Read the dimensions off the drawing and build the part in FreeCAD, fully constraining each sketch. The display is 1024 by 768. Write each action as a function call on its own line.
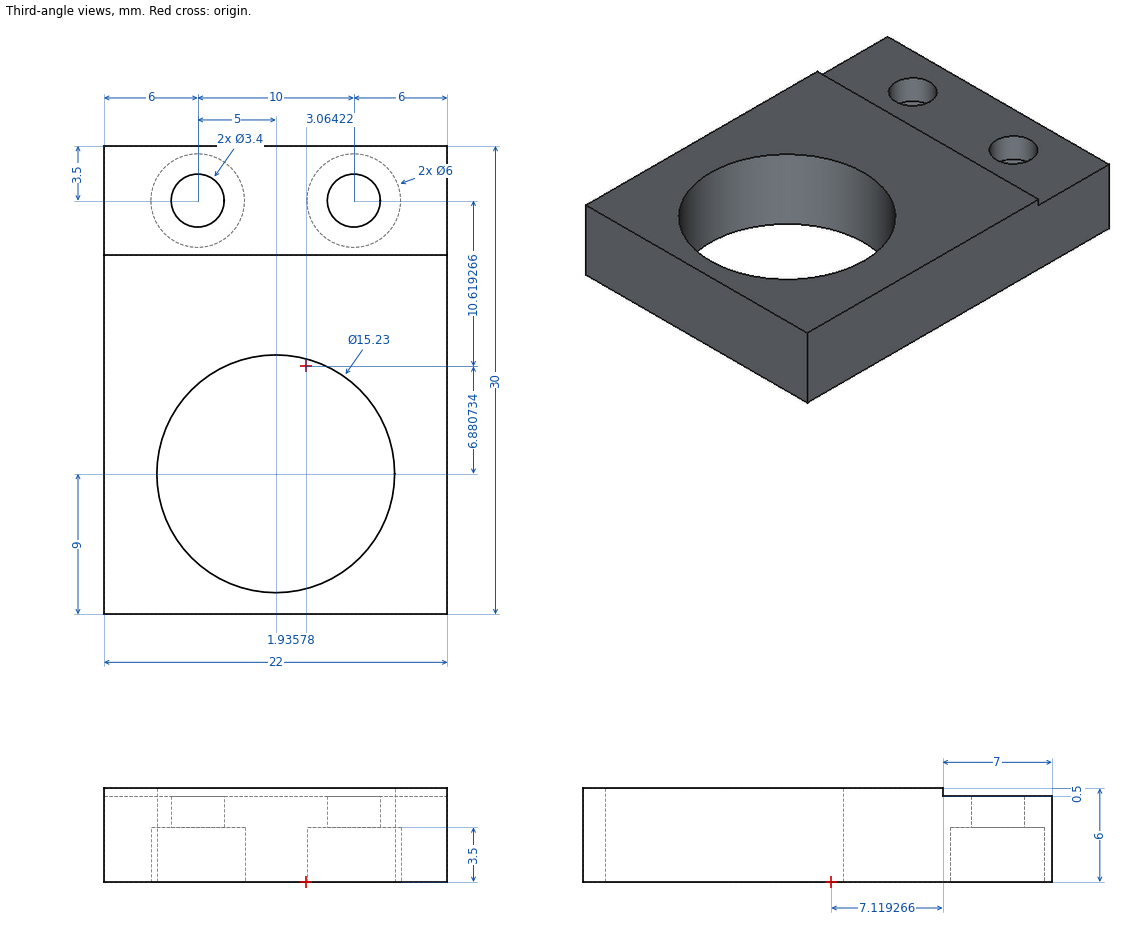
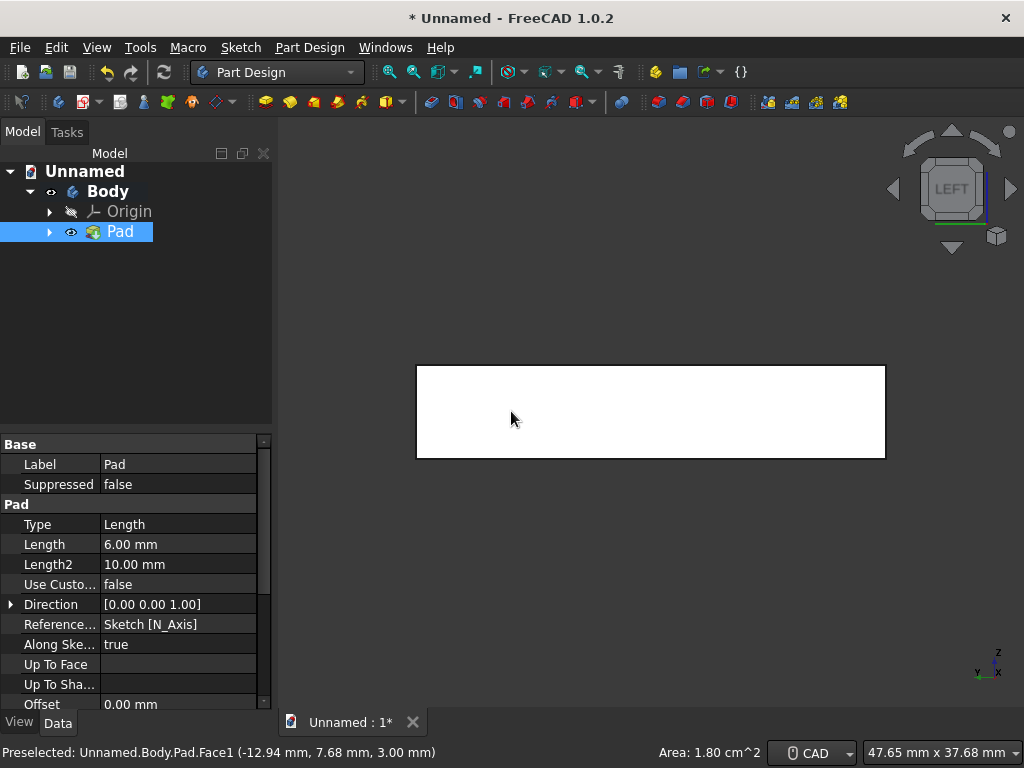
click(84, 102)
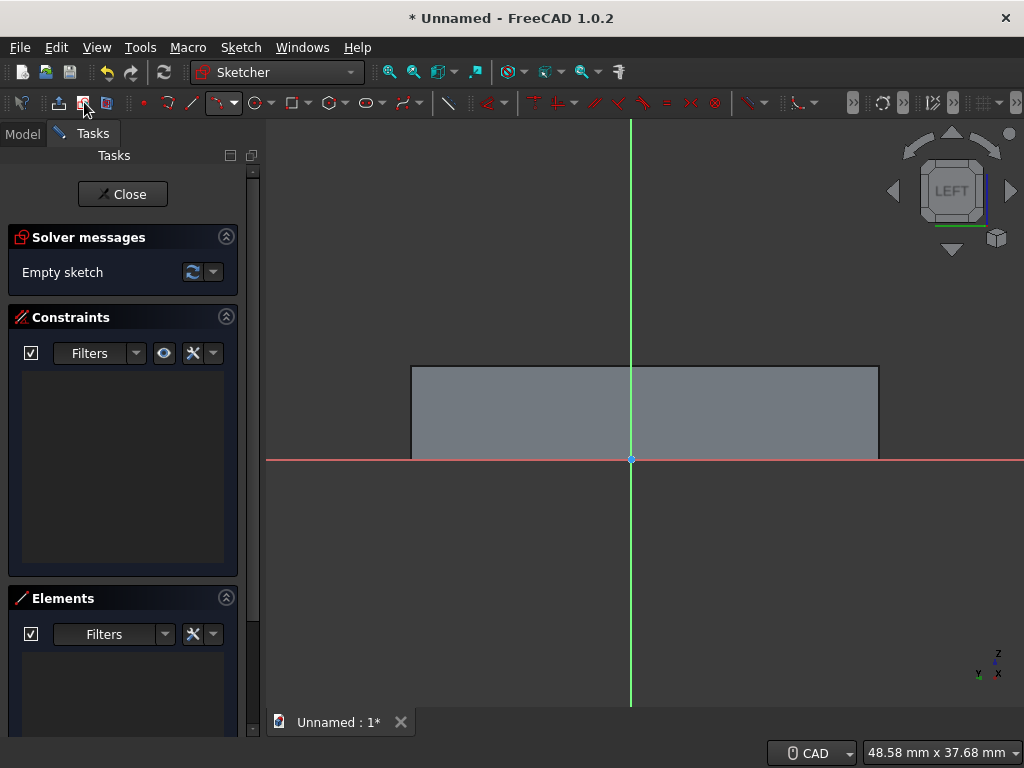
scroll(454, 413, up, 3)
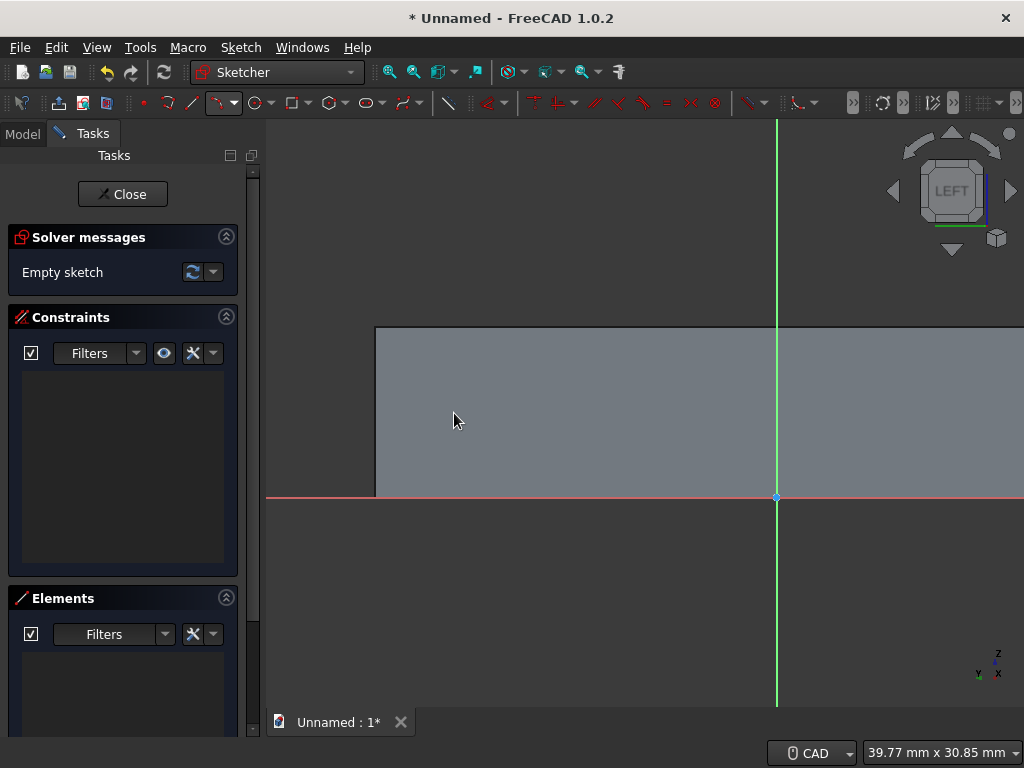
key(g)
key(r)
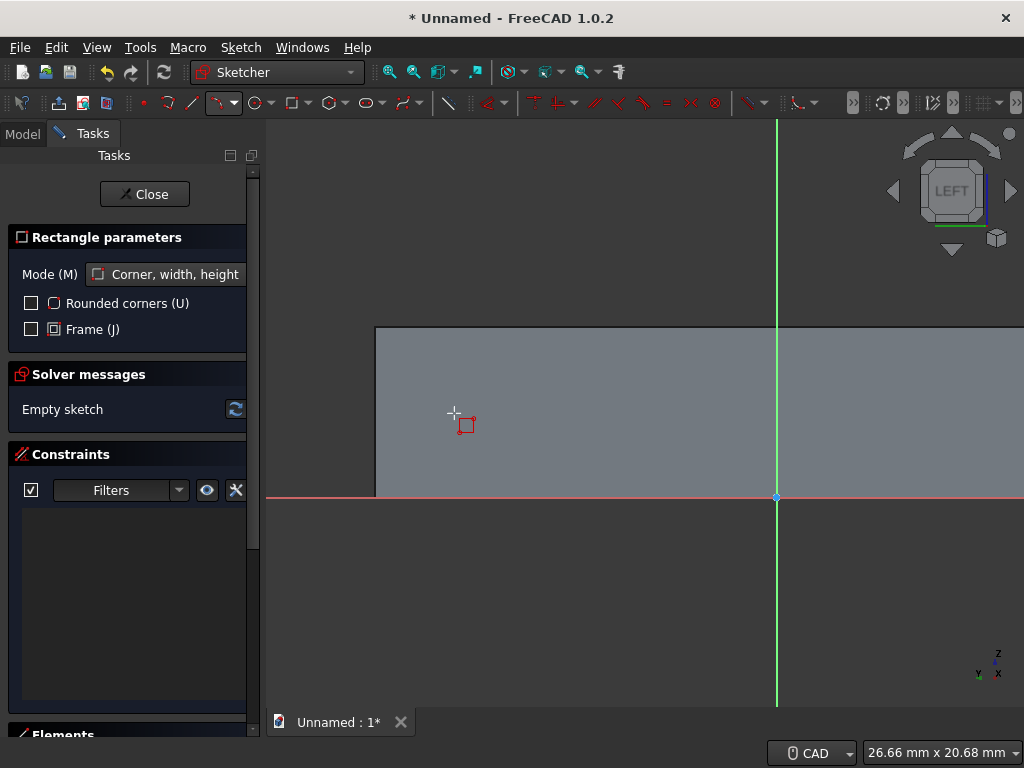
click(375, 327)
move(574, 342)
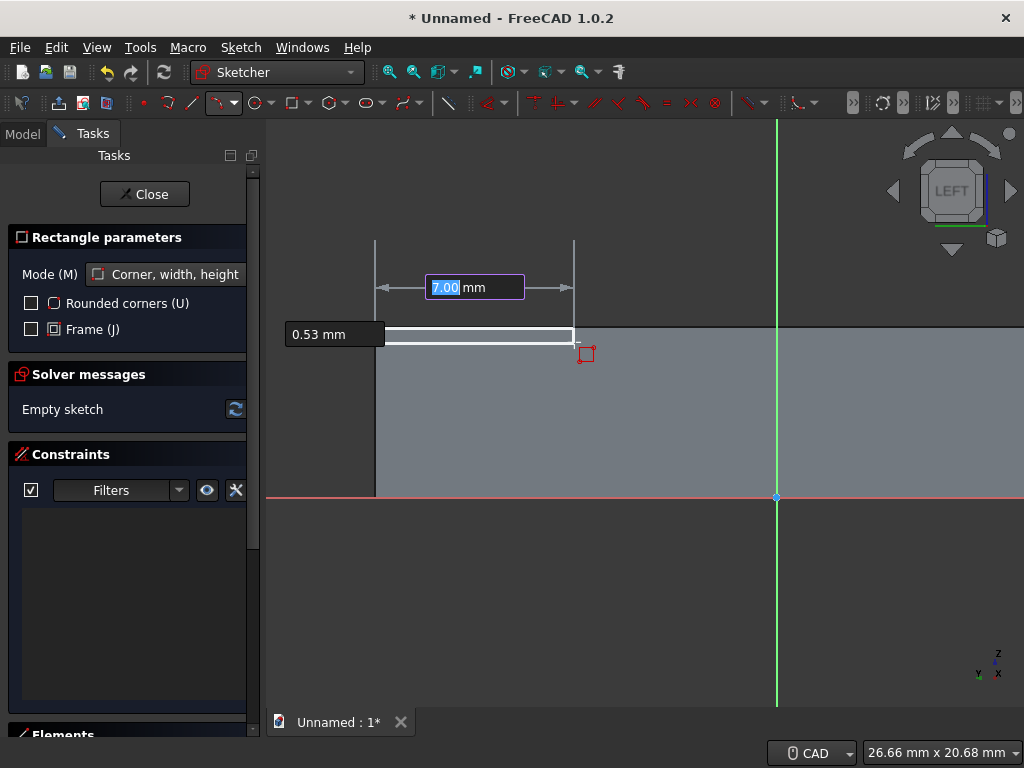
text(7)
key(Tab)
text(0.5)
key(Return)
key(Escape)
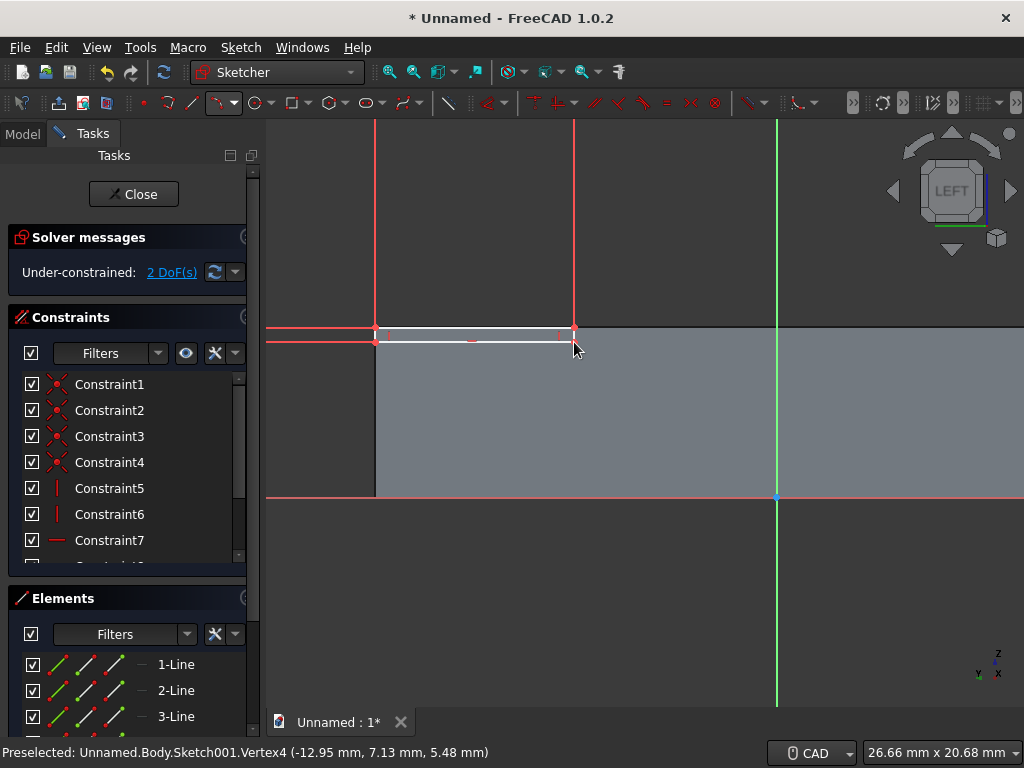
click(375, 328)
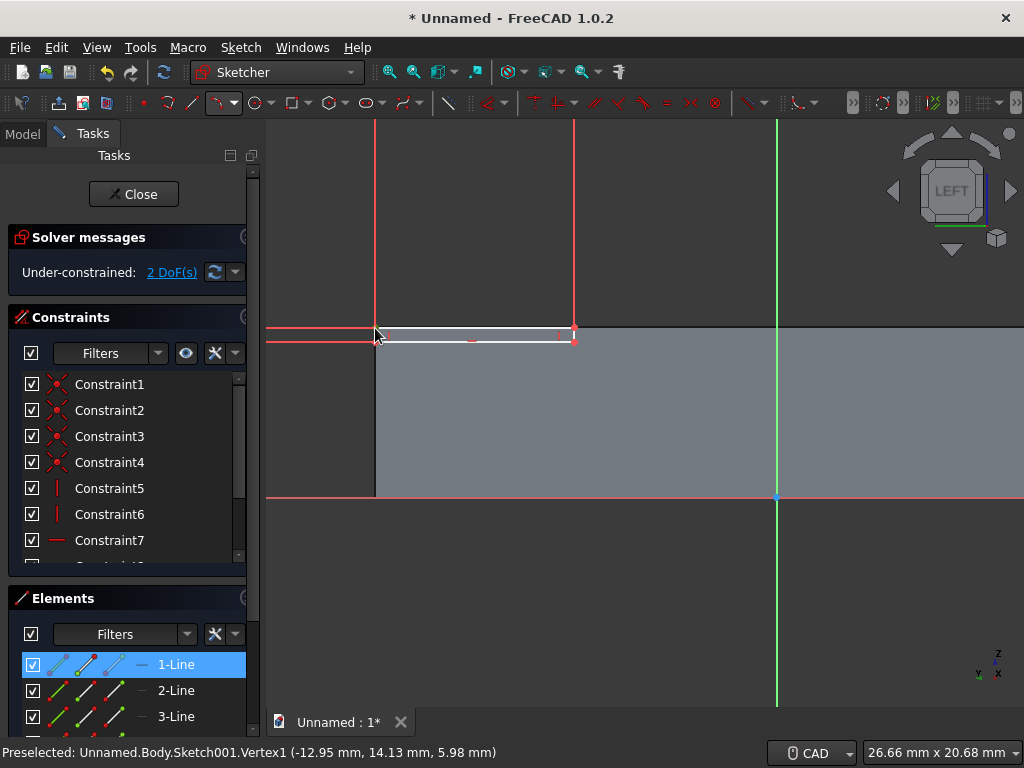
key(i)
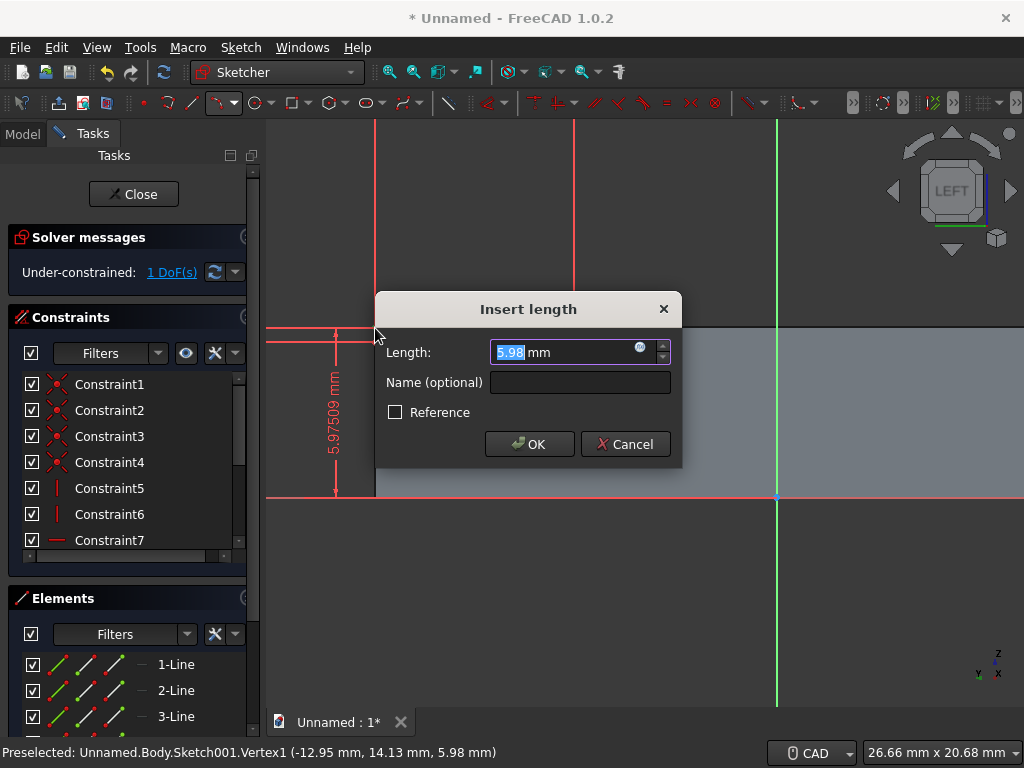
text(6)
key(Return)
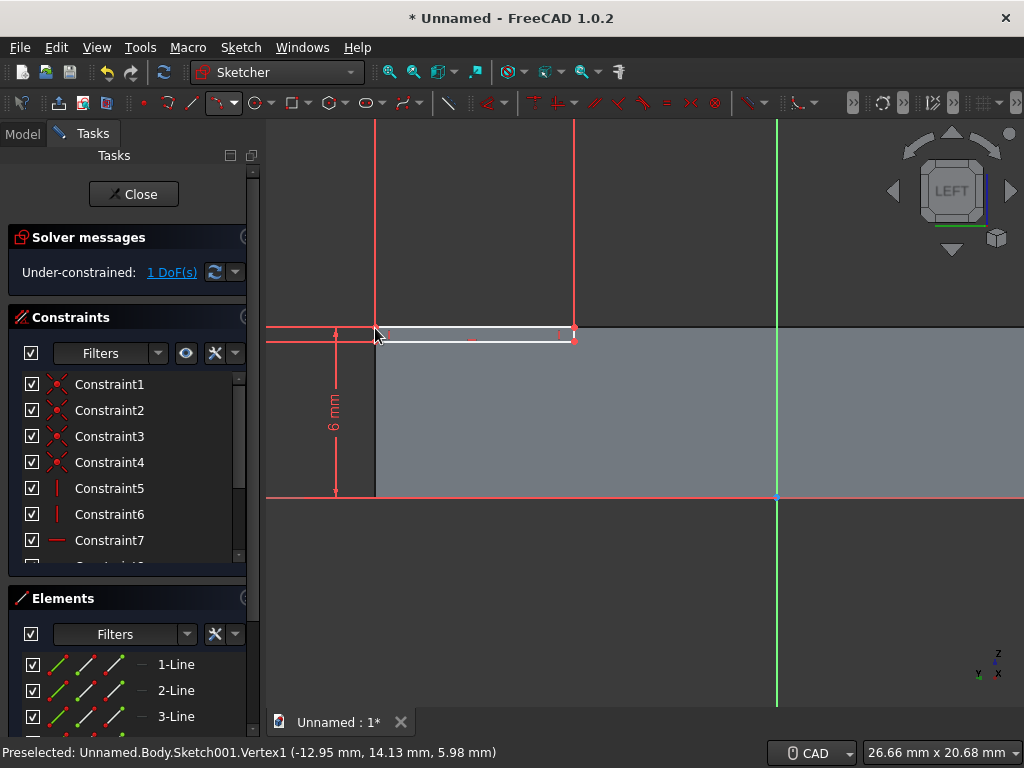
click(574, 342)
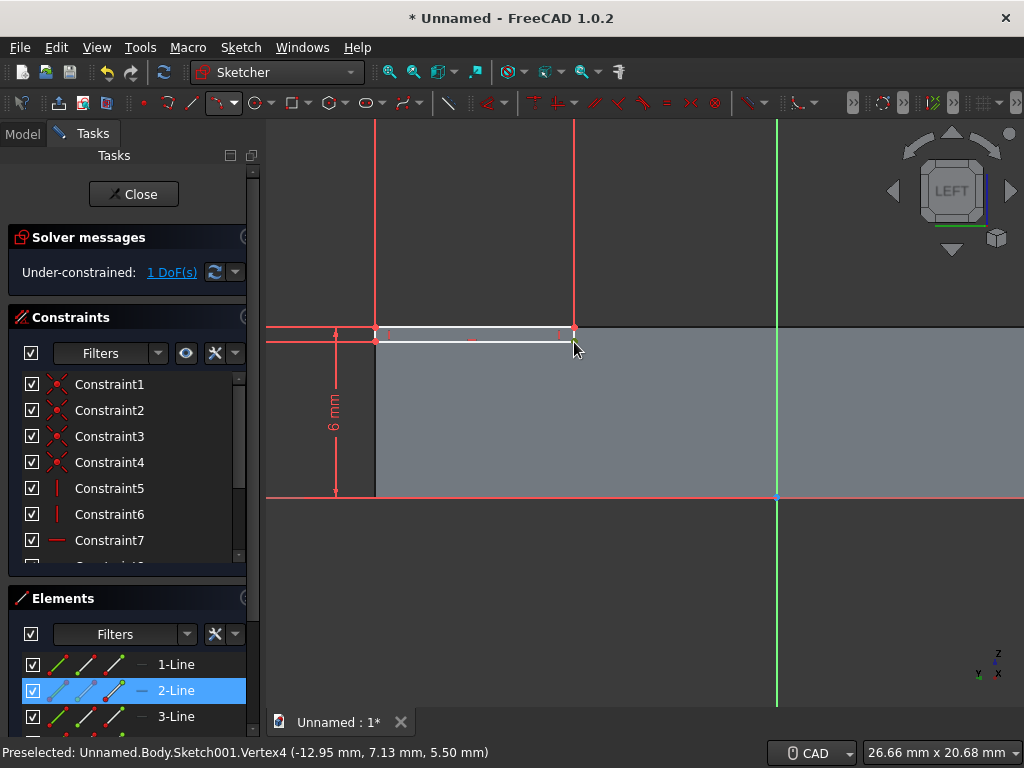
key(l)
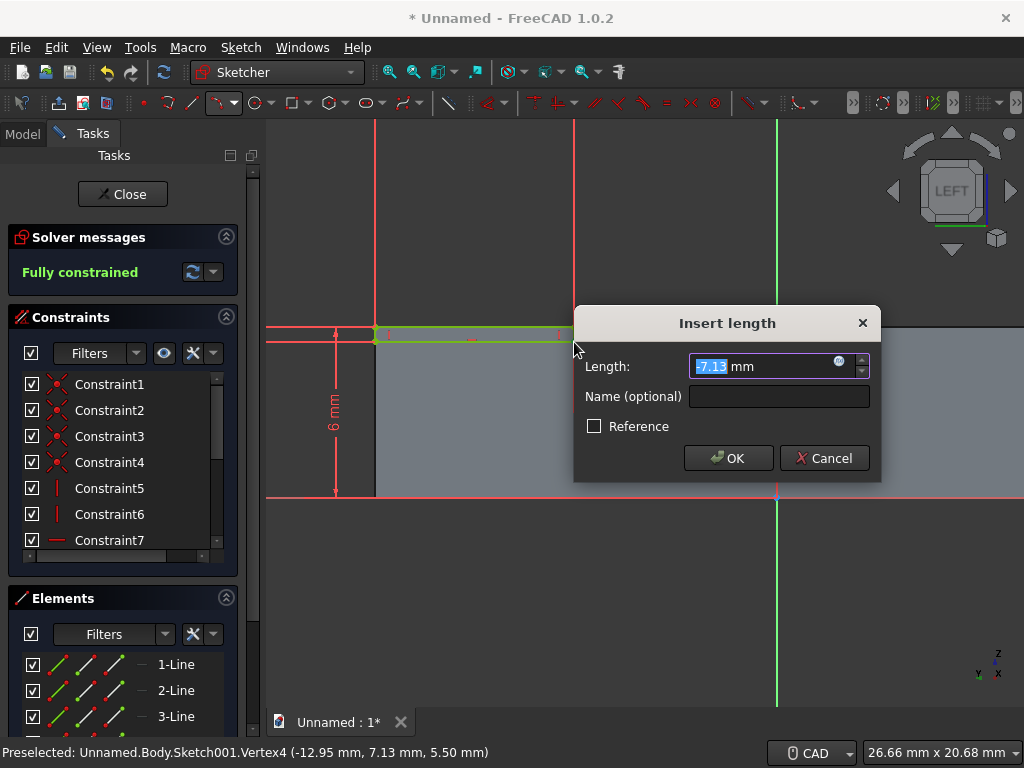
text(-7.119266)
key(Return)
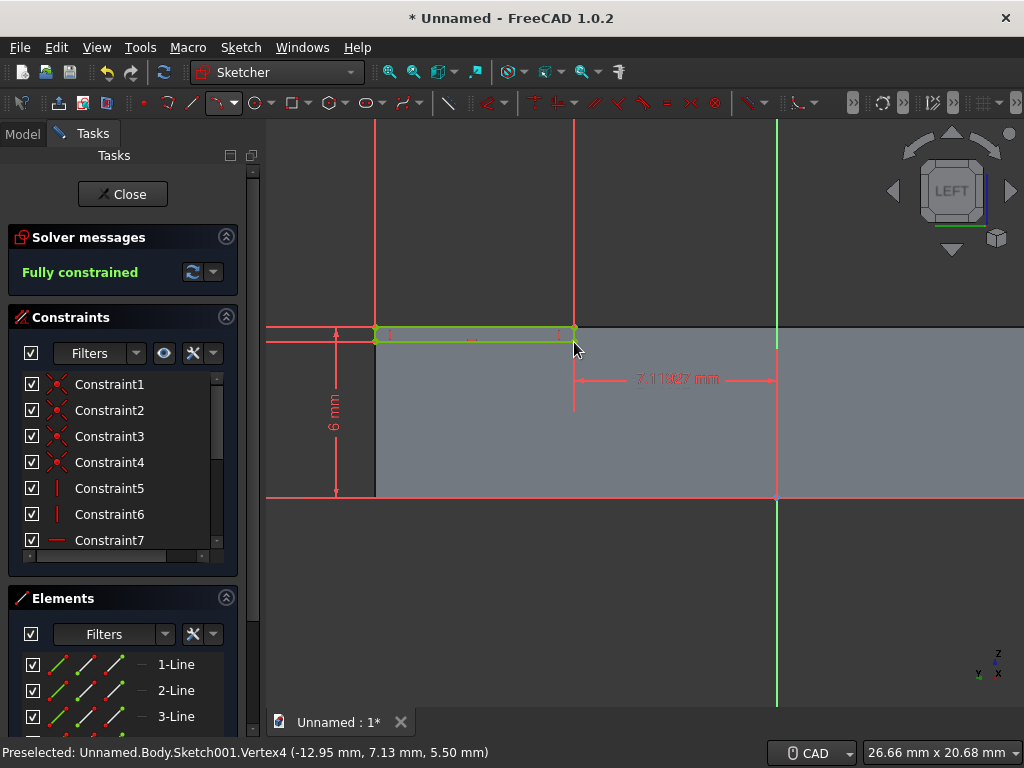
click(123, 194)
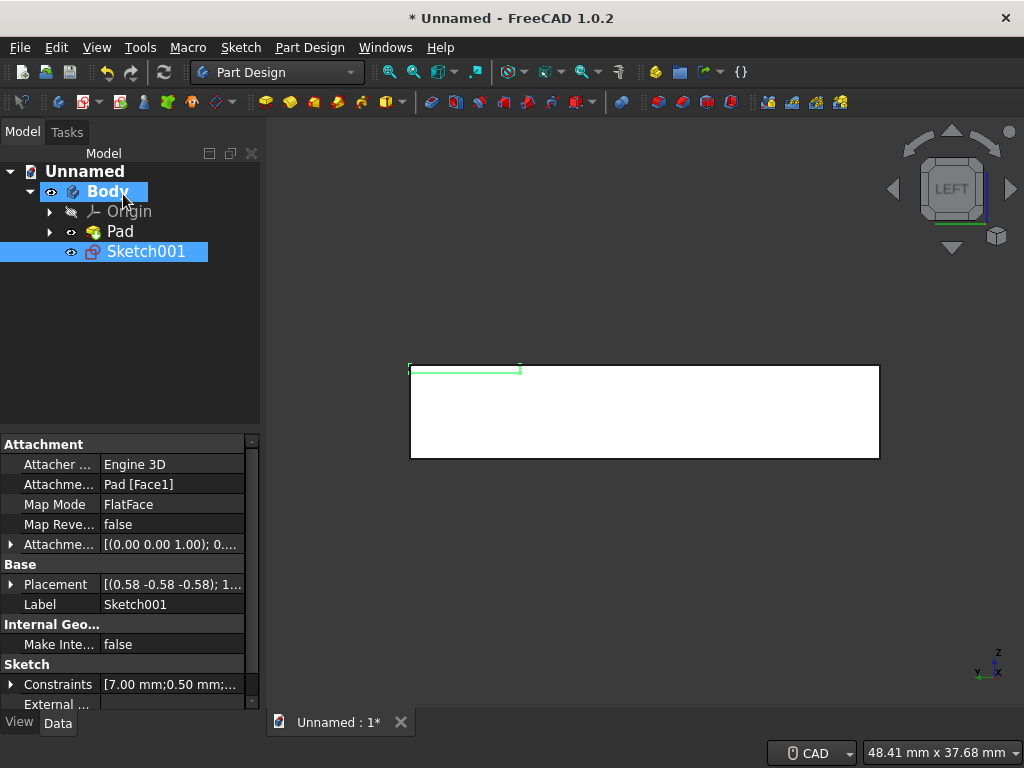
click(432, 102)